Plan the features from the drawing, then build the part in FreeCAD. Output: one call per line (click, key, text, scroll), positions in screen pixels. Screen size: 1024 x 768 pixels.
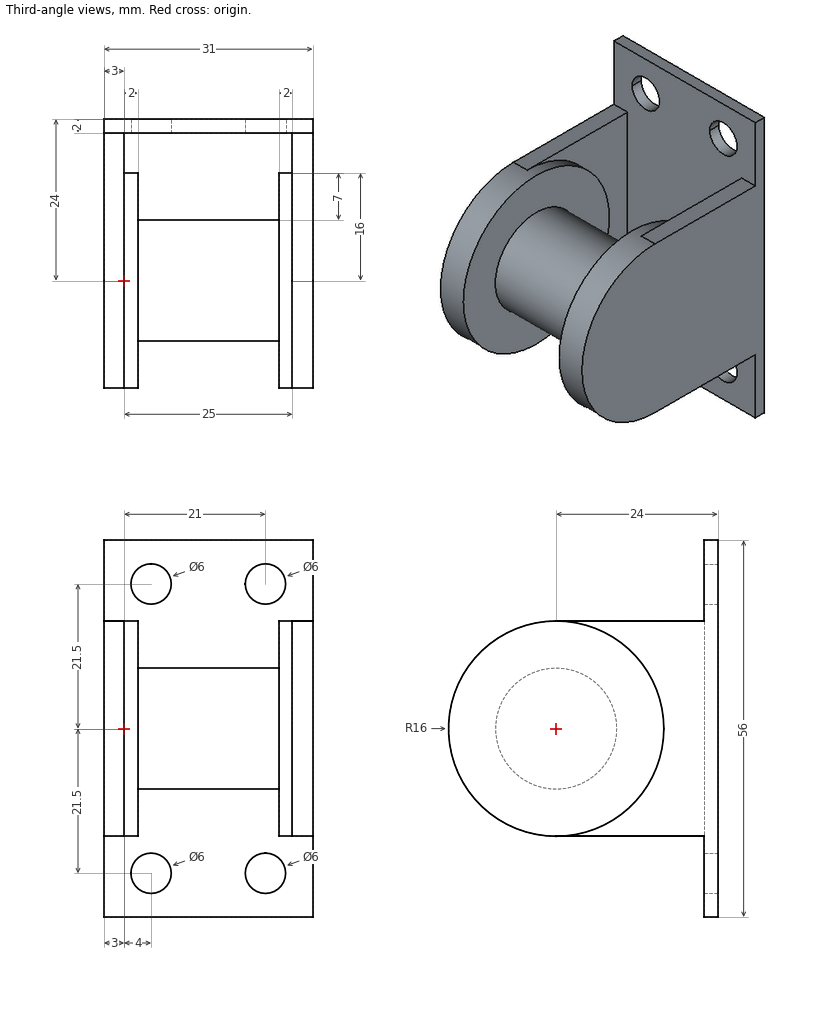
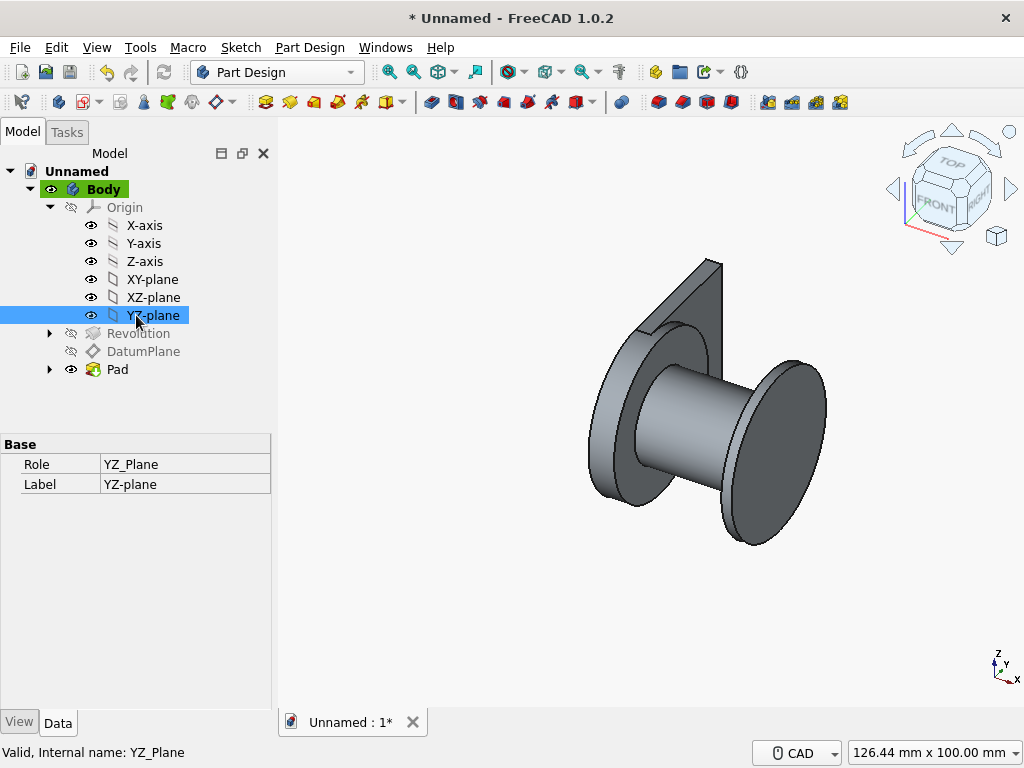
click(216, 102)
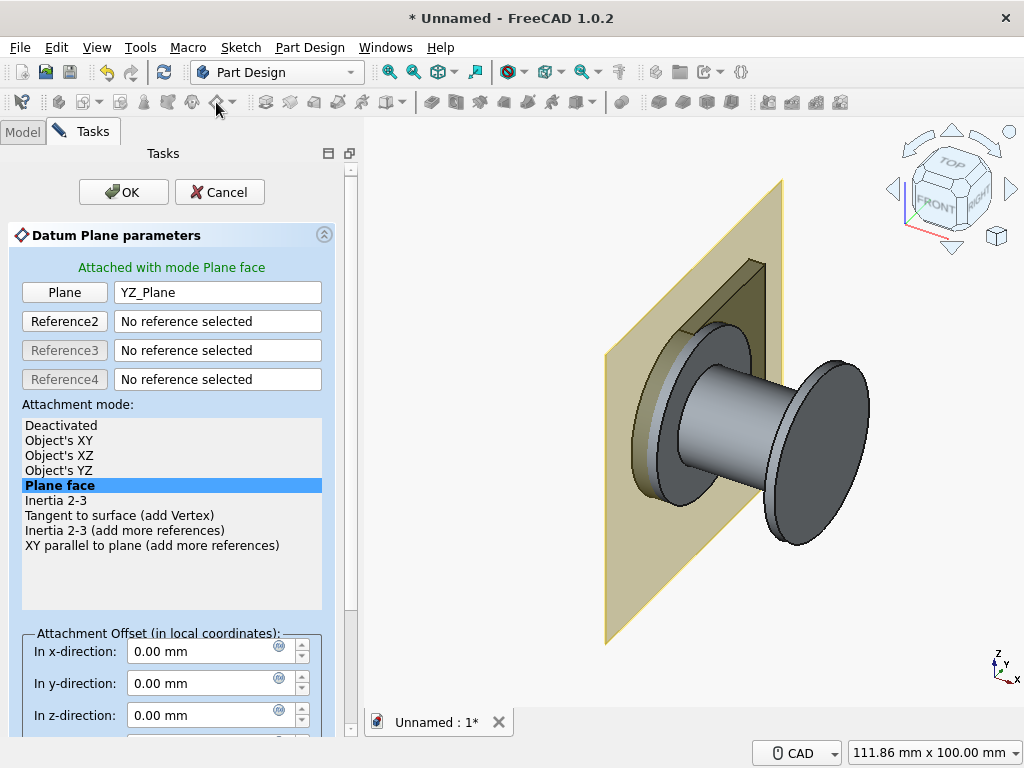
triple_click(210, 715)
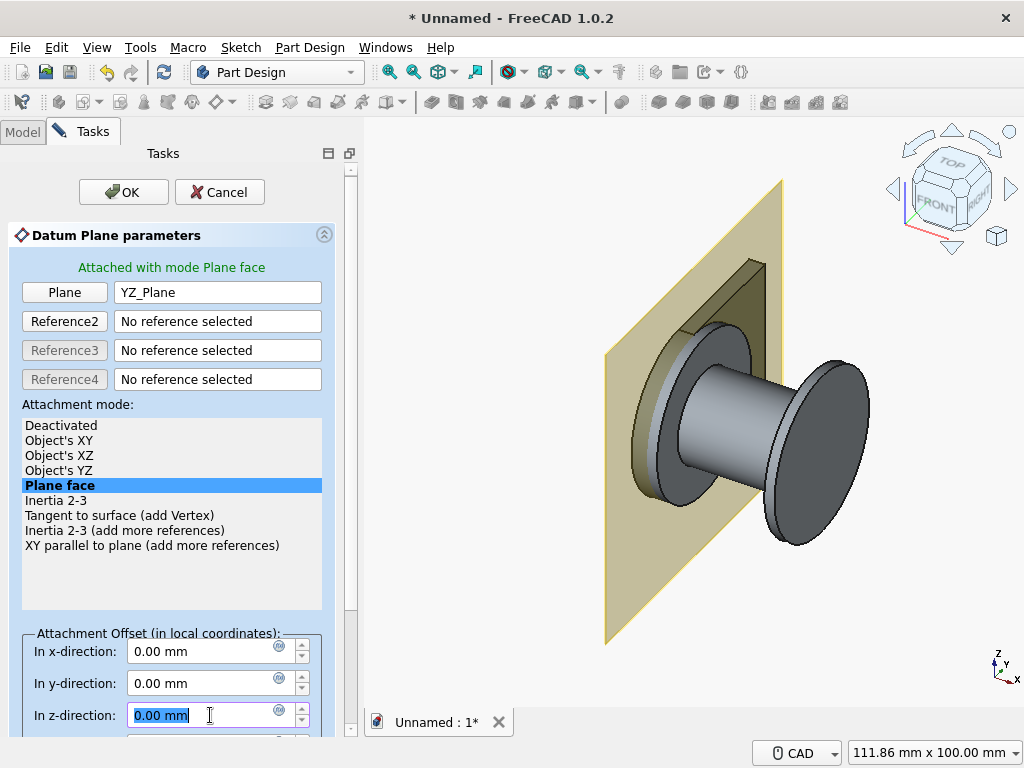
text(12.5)
key(Tab)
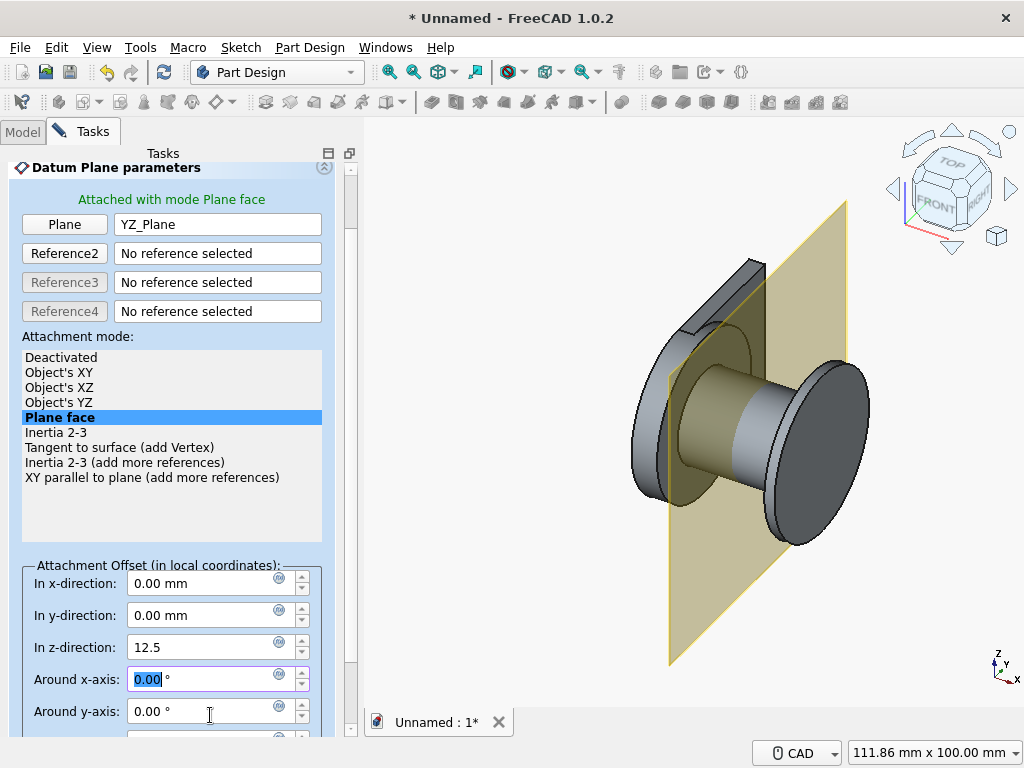
scroll(351, 450, up, 2)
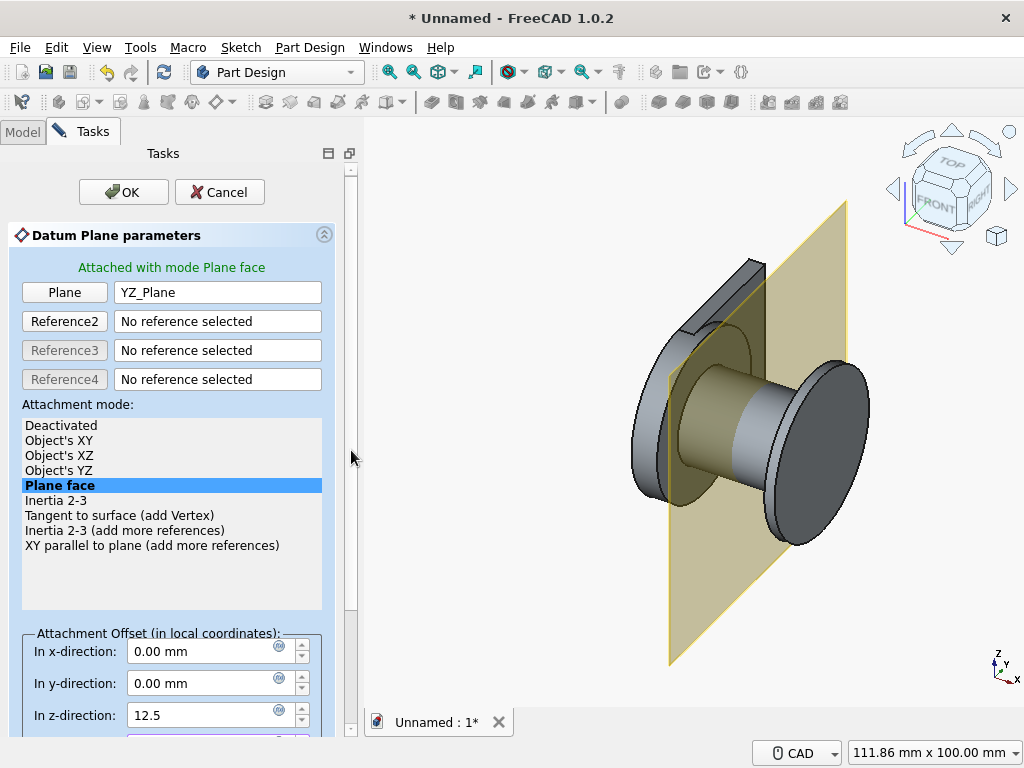
click(124, 192)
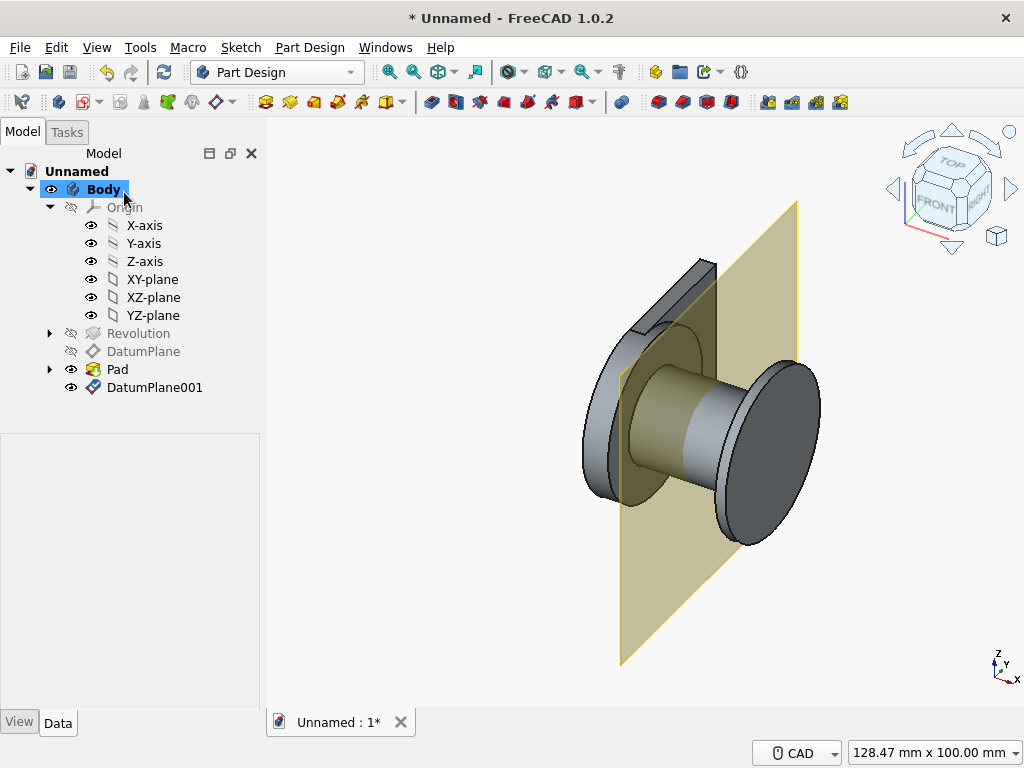
click(116, 369)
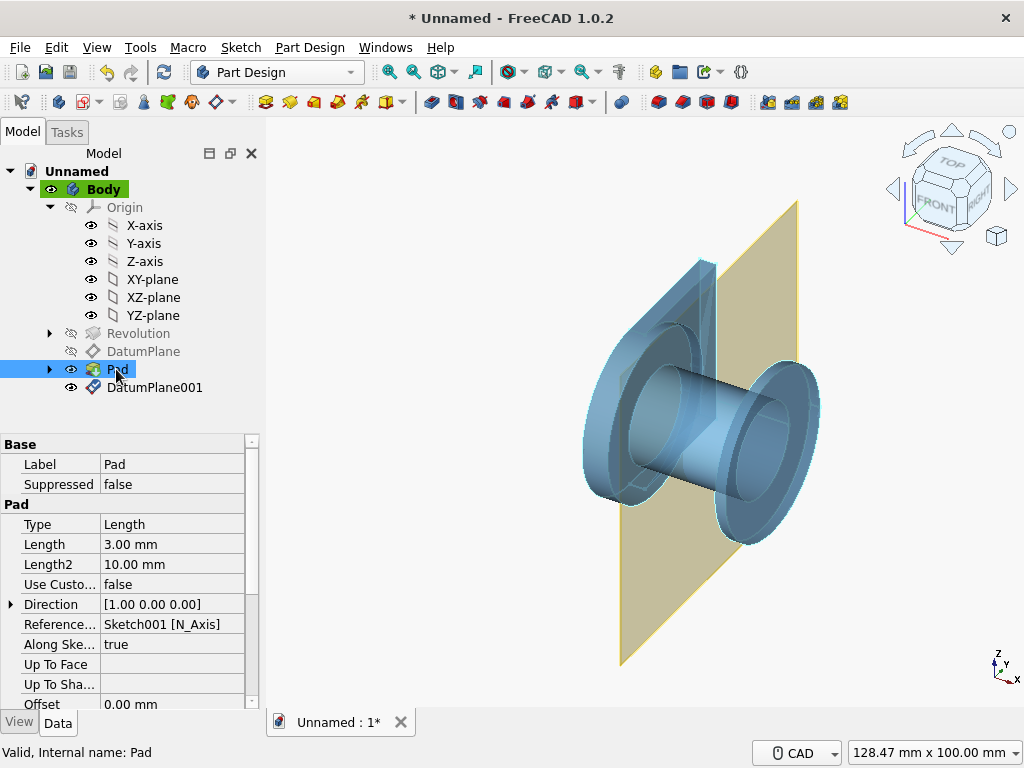
click(768, 102)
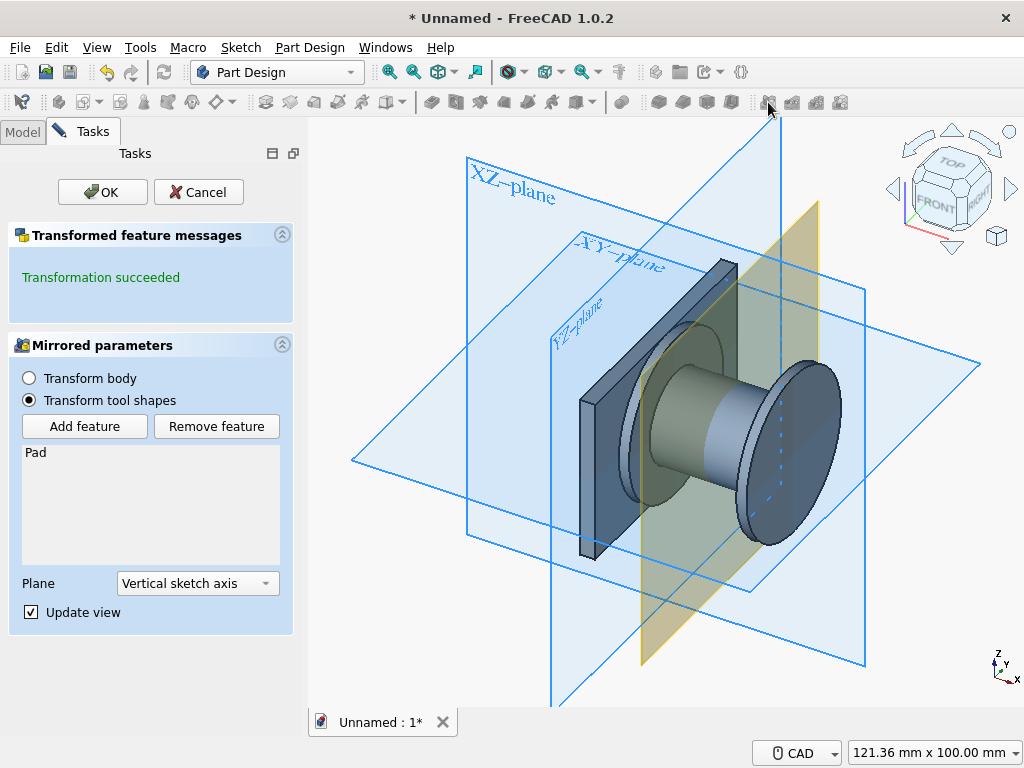
click(198, 584)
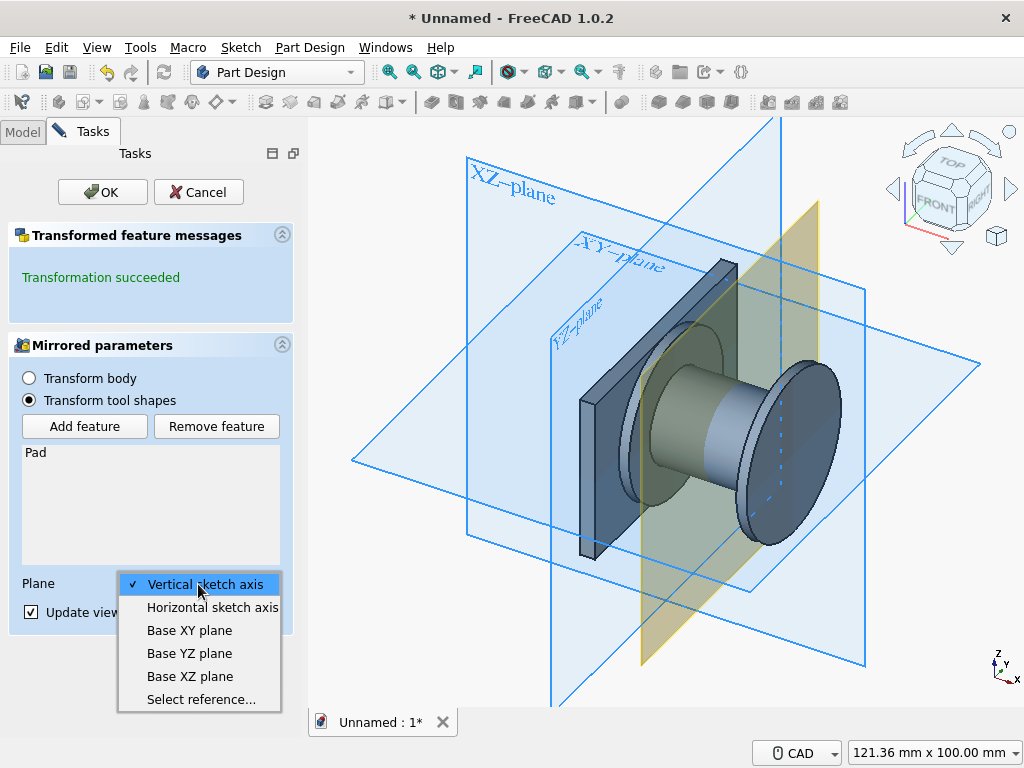
click(198, 700)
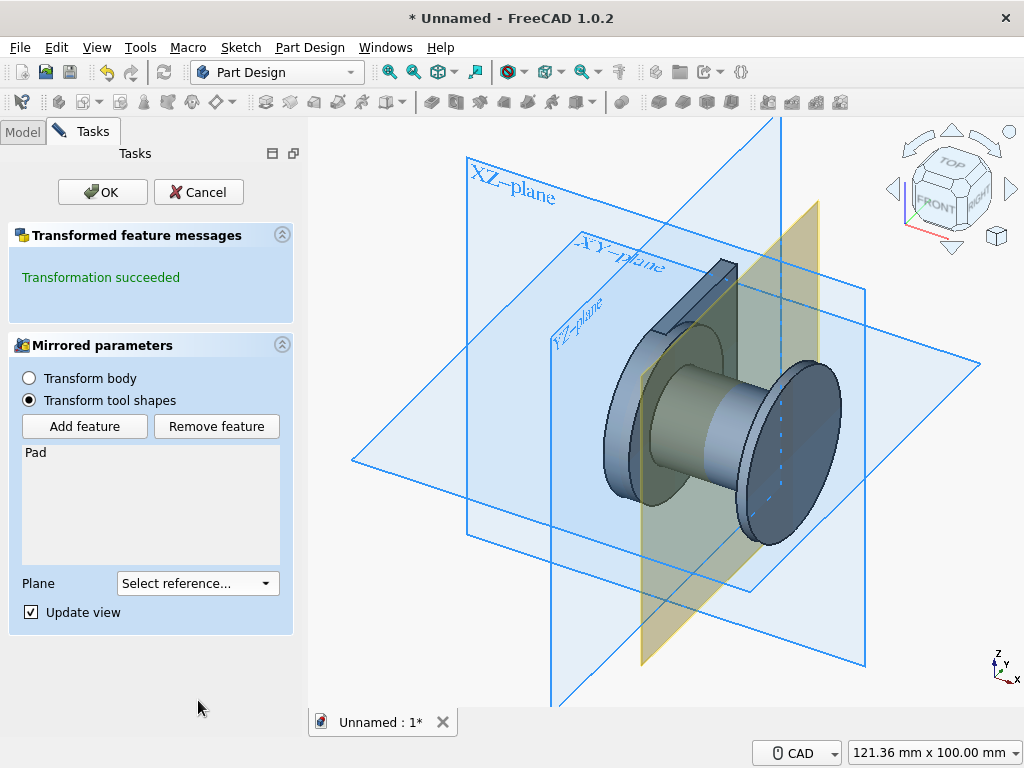
click(23, 131)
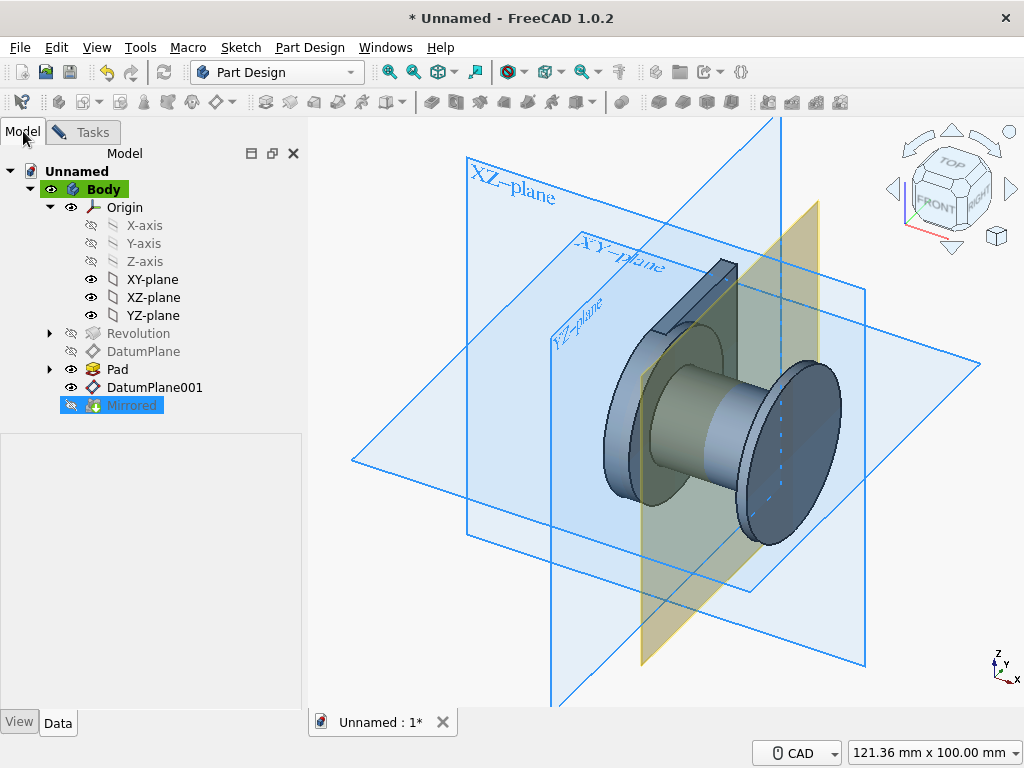
click(116, 387)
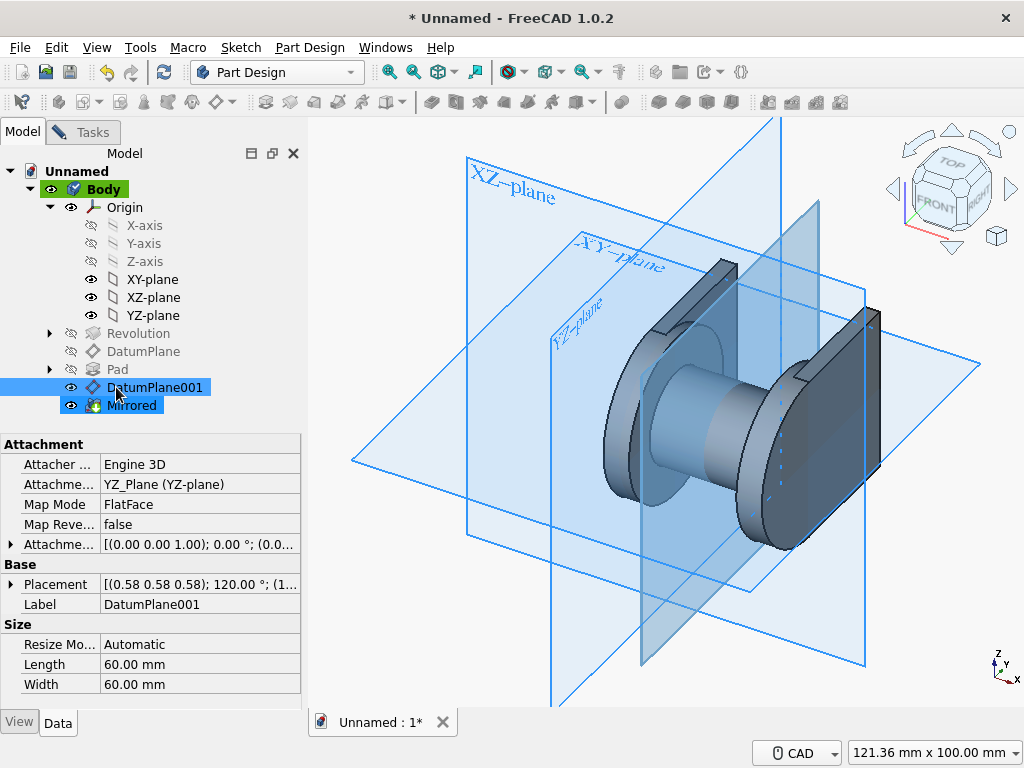
click(84, 131)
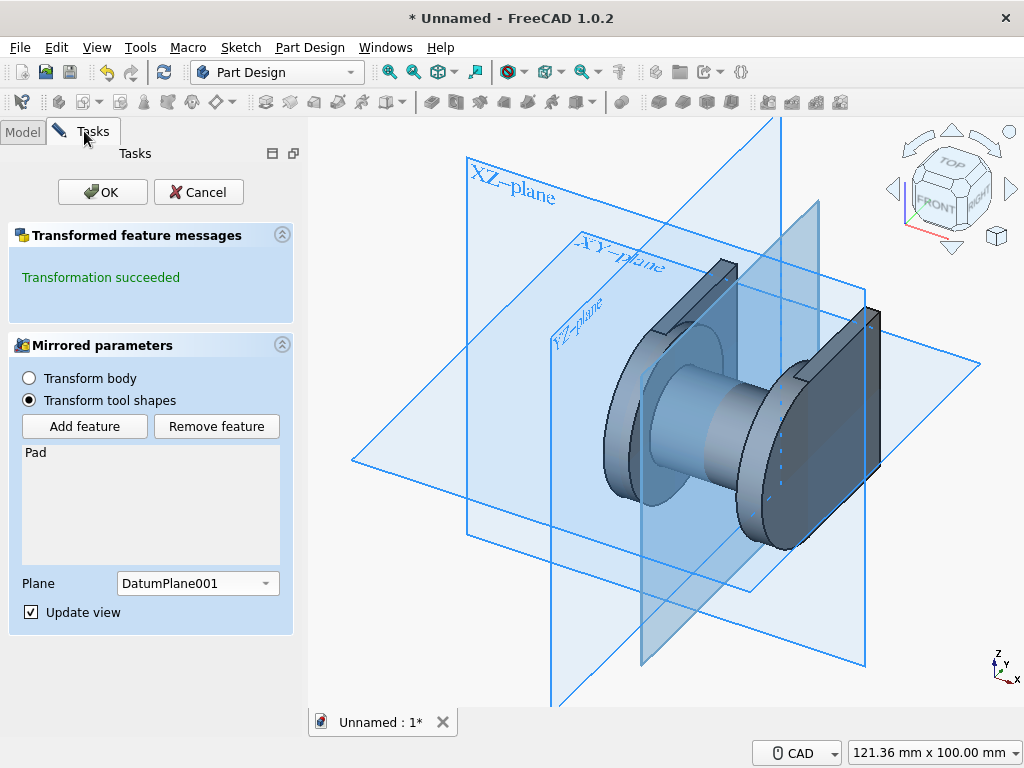
click(103, 192)